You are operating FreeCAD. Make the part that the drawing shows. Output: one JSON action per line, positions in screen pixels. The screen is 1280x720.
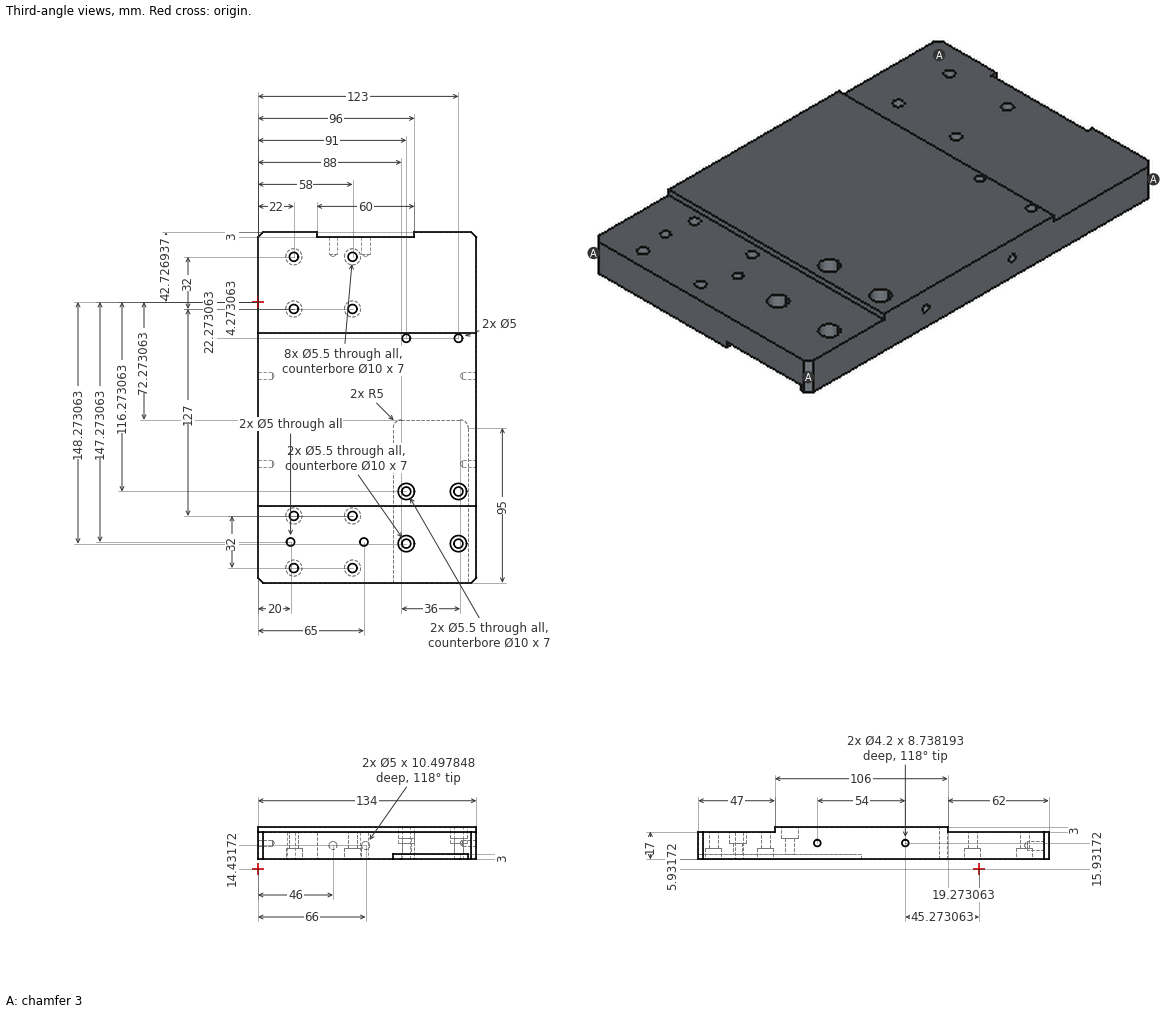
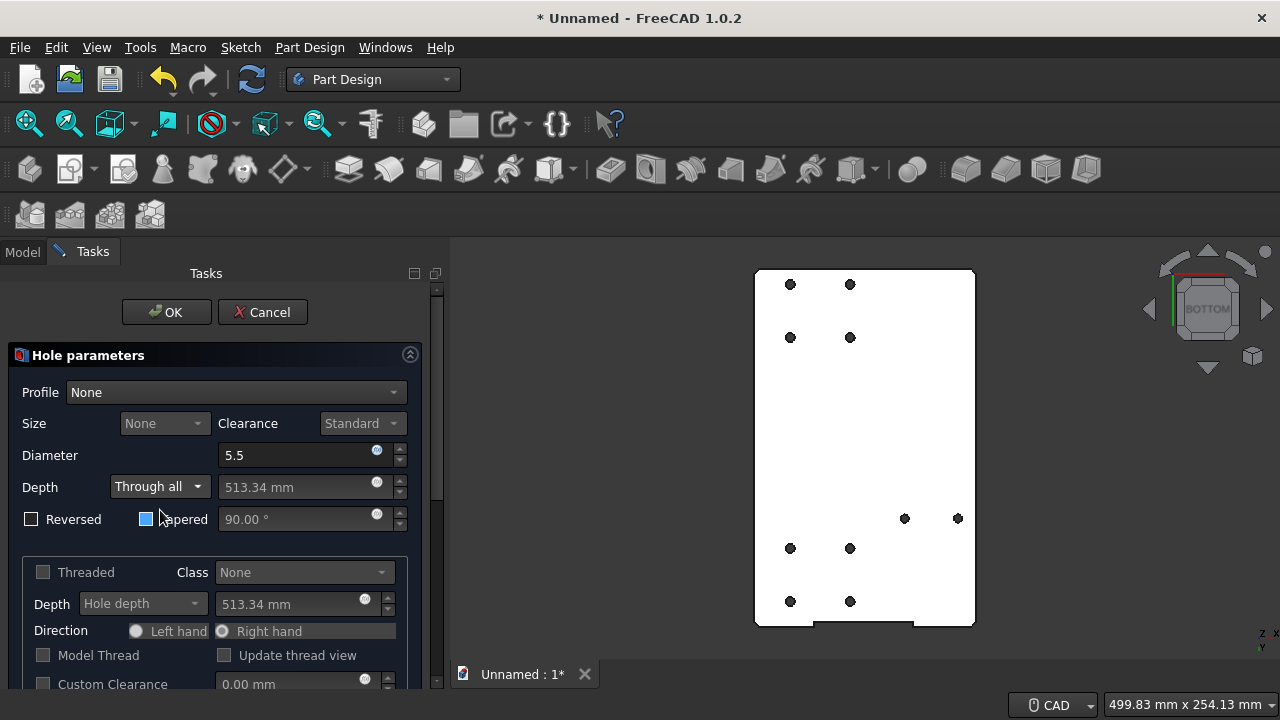
{"action": "scroll", "coordinate": [437, 486], "scroll_direction": "down", "scroll_amount": 3}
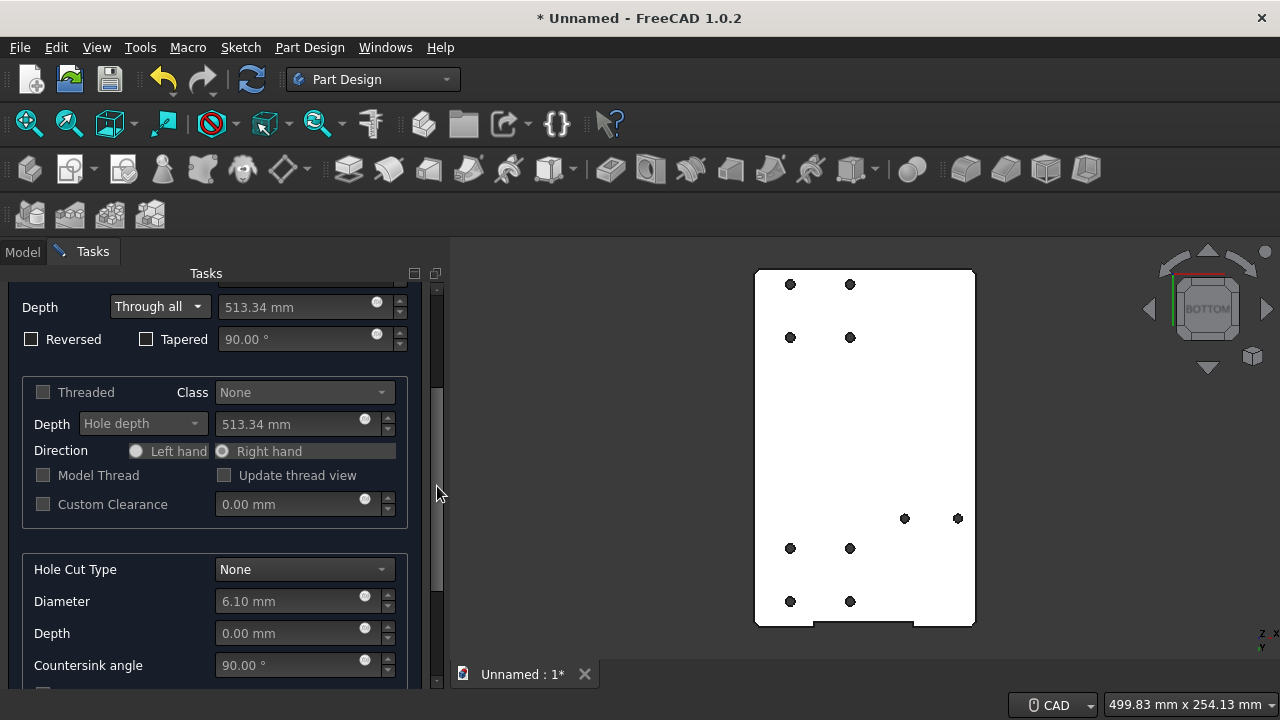
{"action": "left_click", "coordinate": [306, 570]}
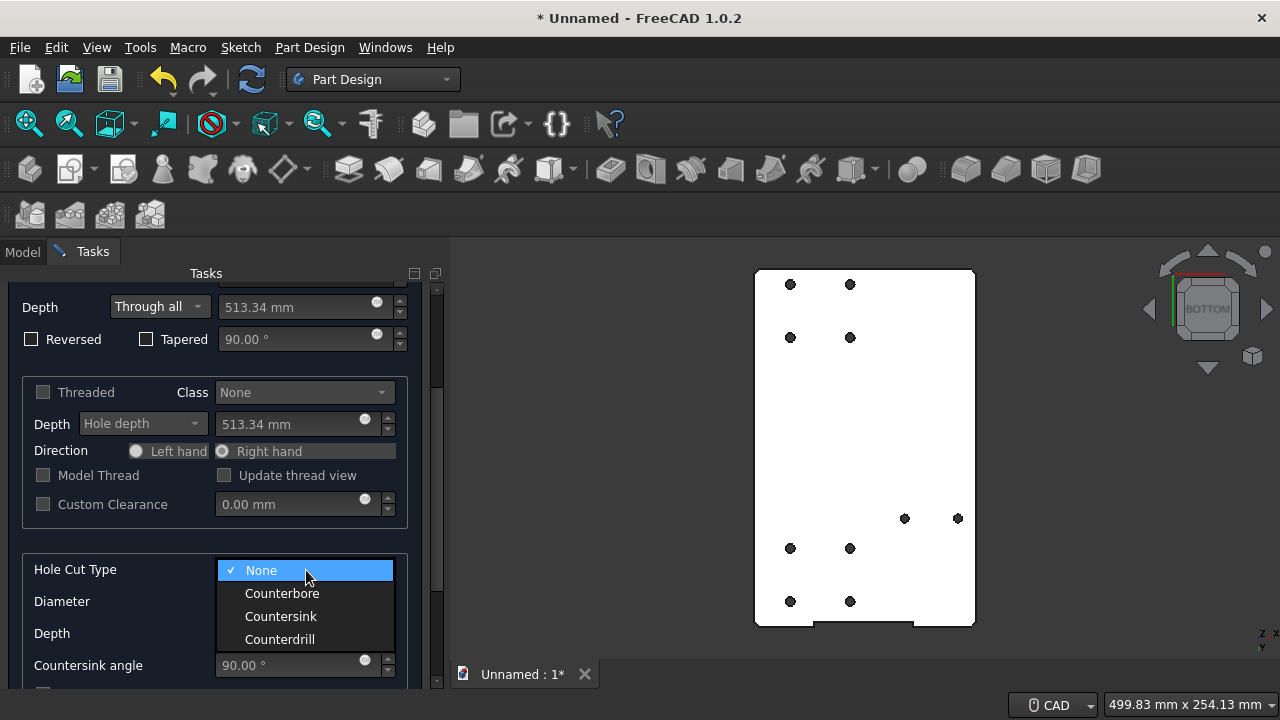
{"action": "left_click", "coordinate": [304, 594]}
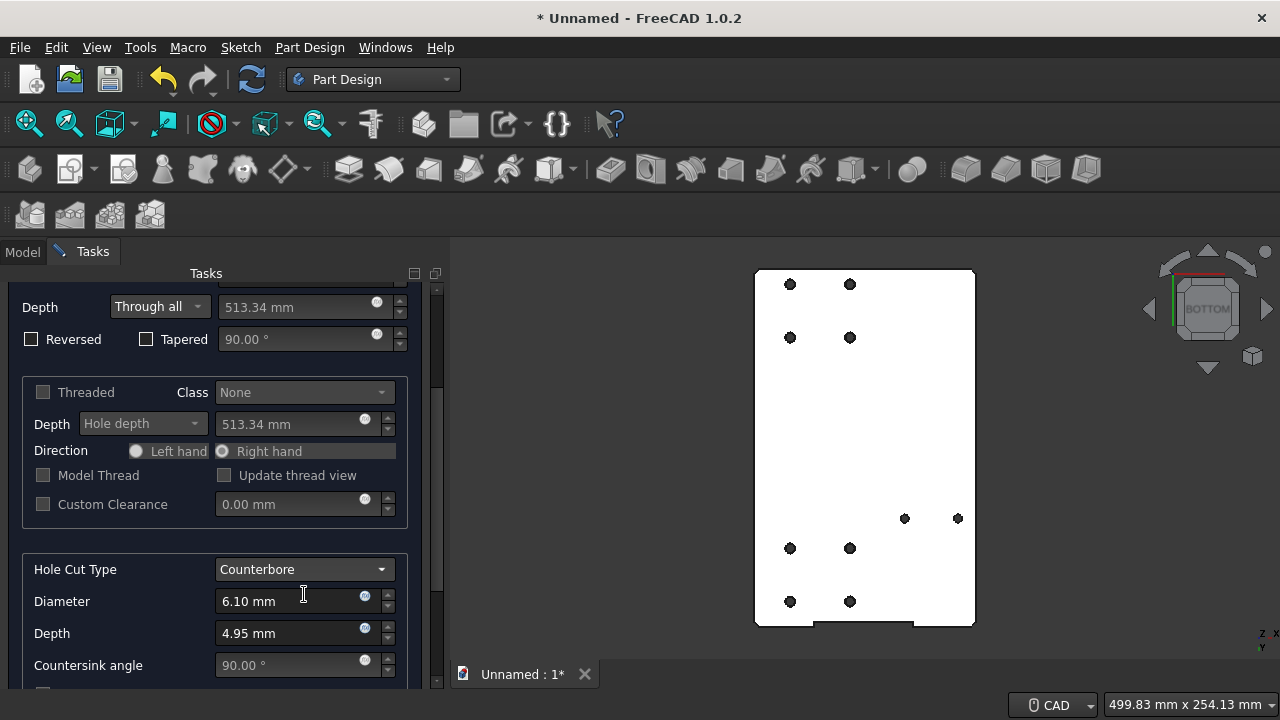
{"action": "triple_click", "coordinate": [298, 601]}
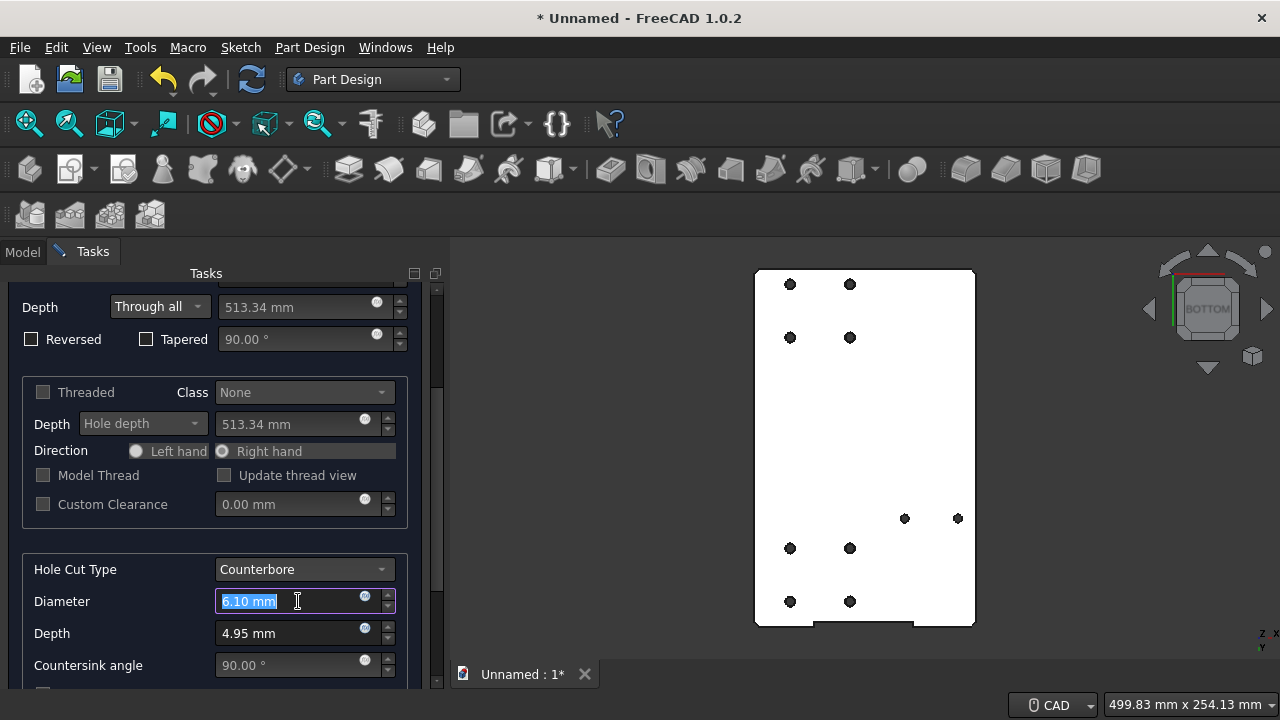
{"action": "type", "text": "10"}
{"action": "key", "text": "Tab"}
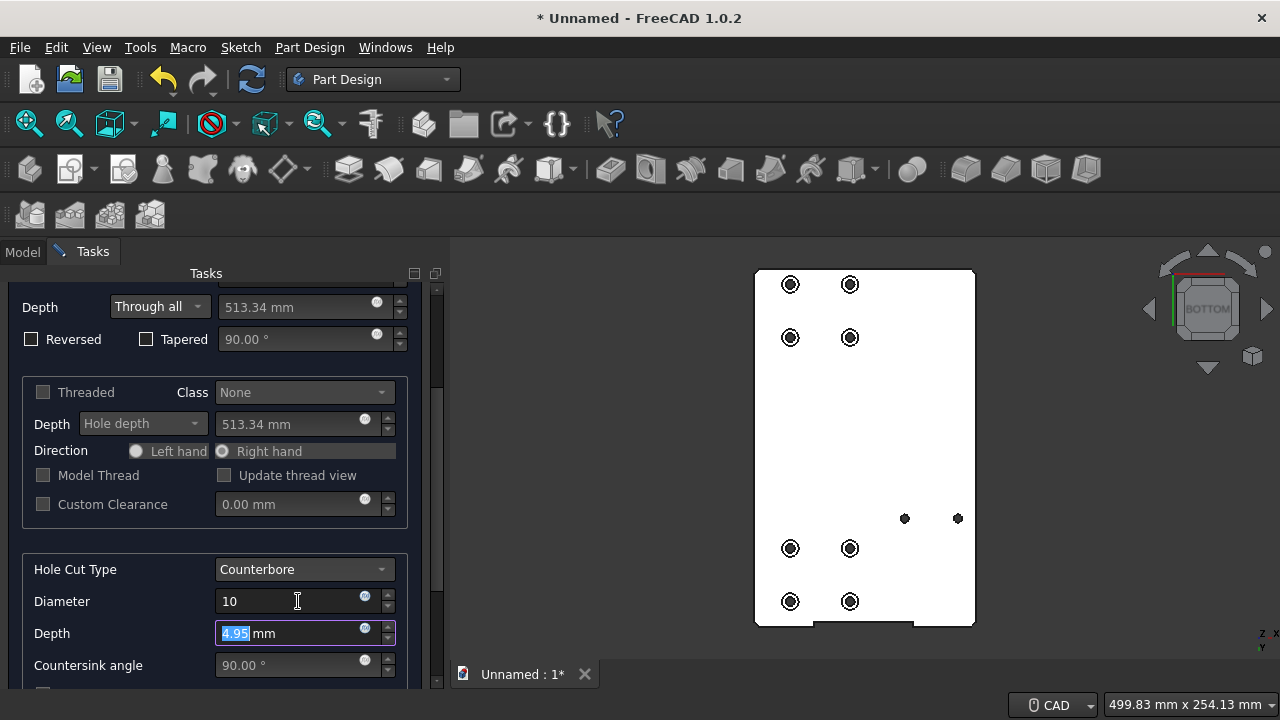
{"action": "type", "text": "7"}
{"action": "key", "text": "Tab"}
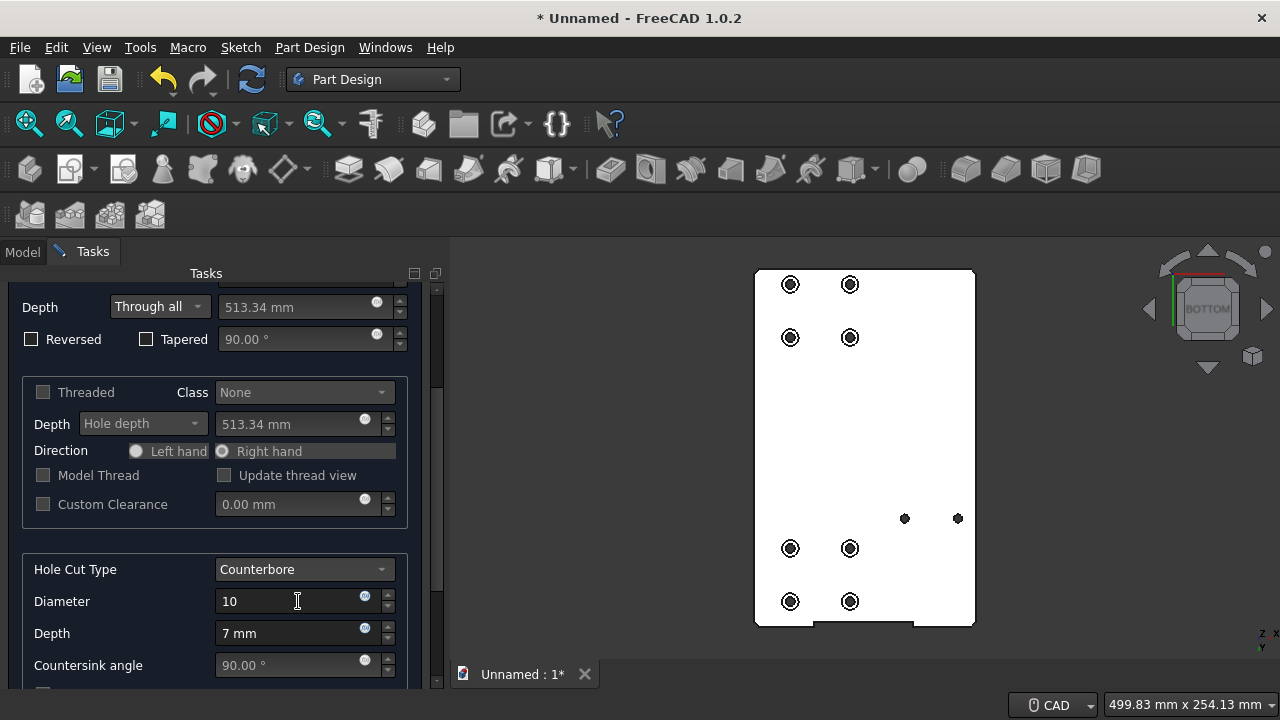
{"action": "scroll", "coordinate": [437, 486], "scroll_direction": "up", "scroll_amount": 4}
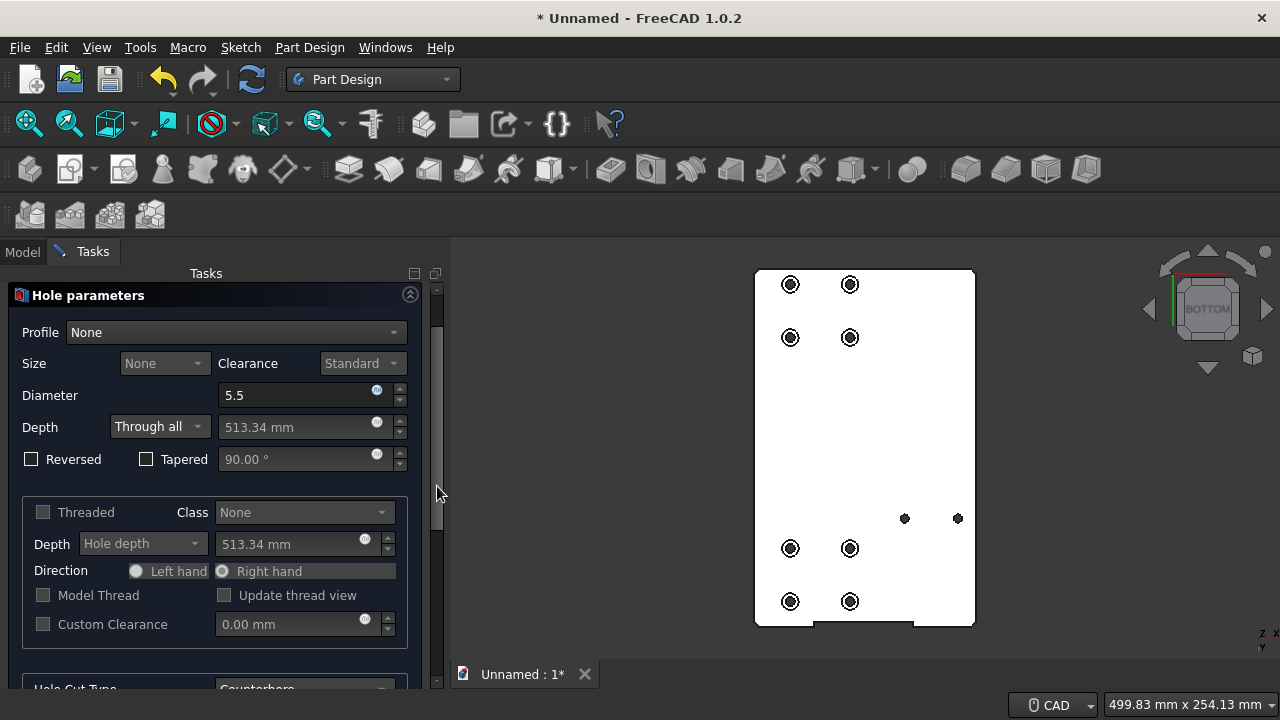
{"action": "left_click", "coordinate": [167, 312]}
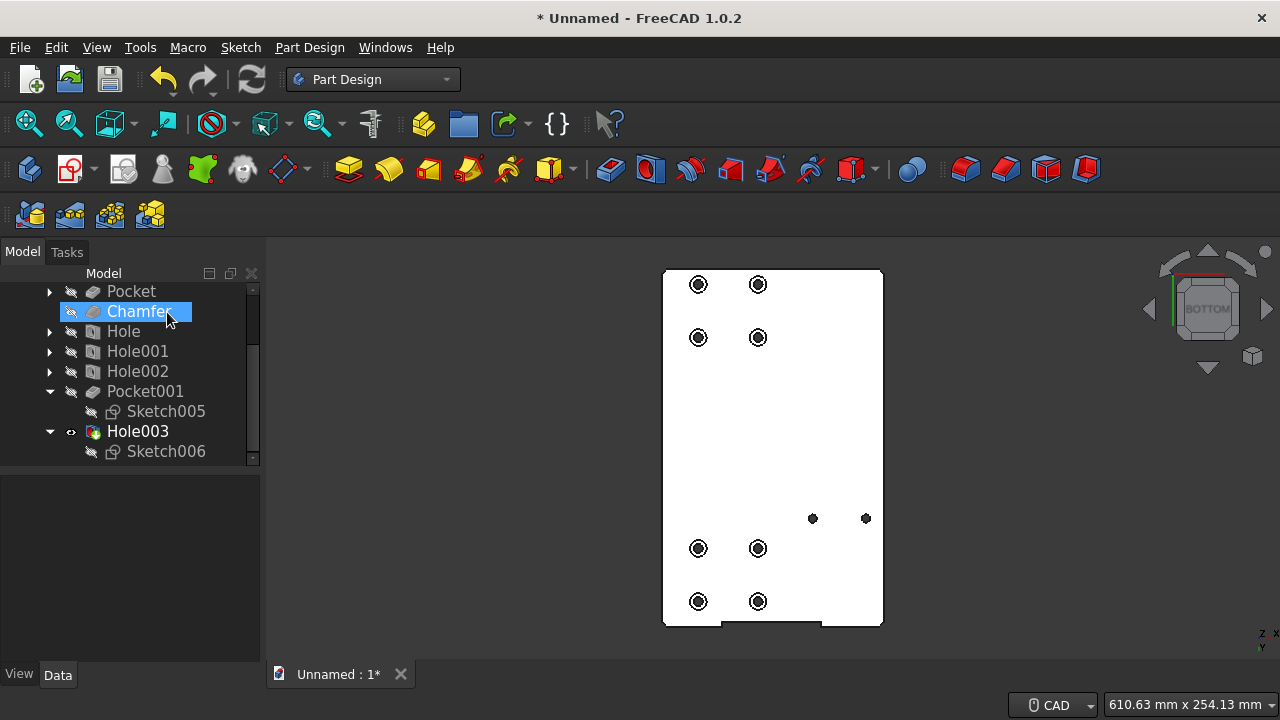
{"action": "left_click", "coordinate": [741, 447]}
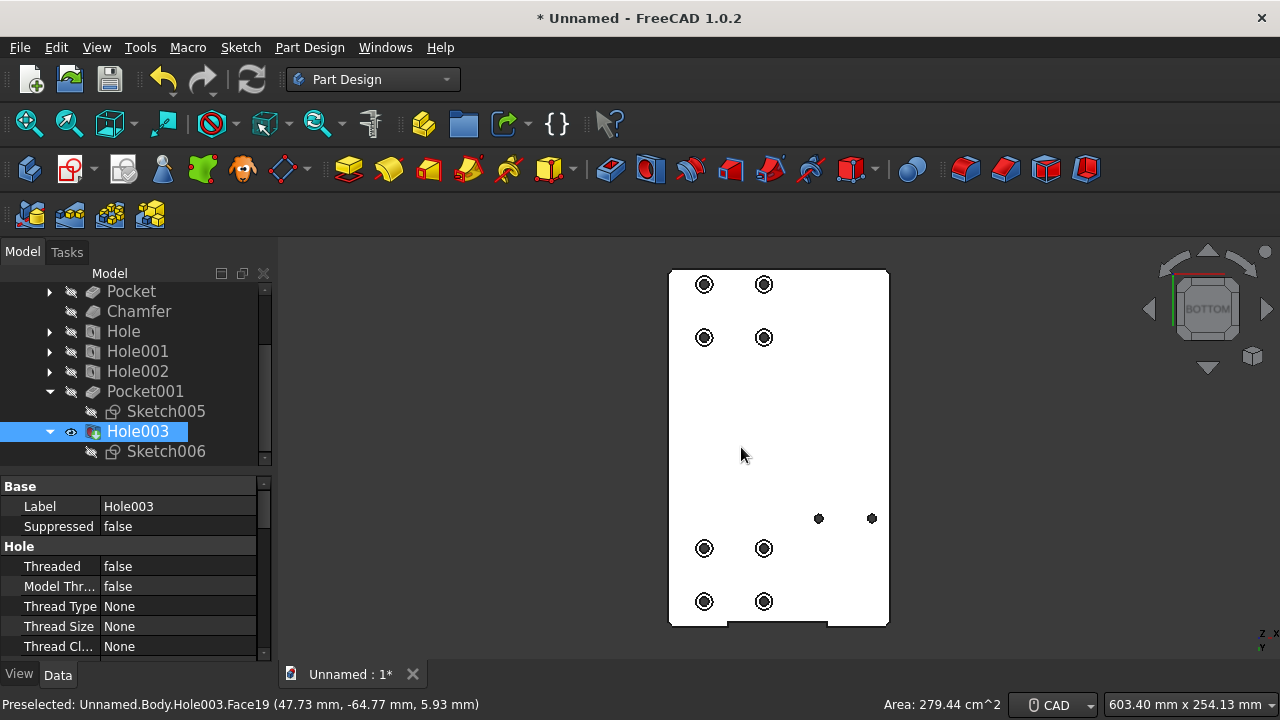
{"action": "left_click", "coordinate": [70, 170]}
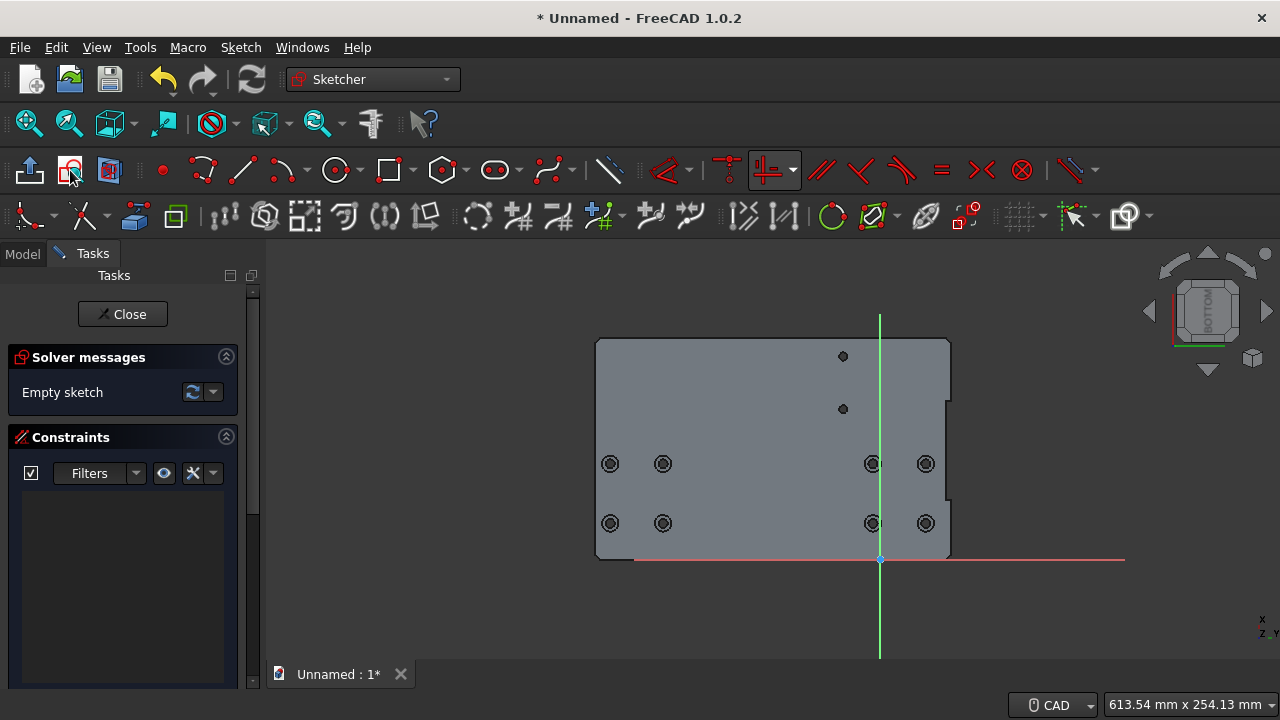
{"action": "left_click", "coordinate": [244, 170]}